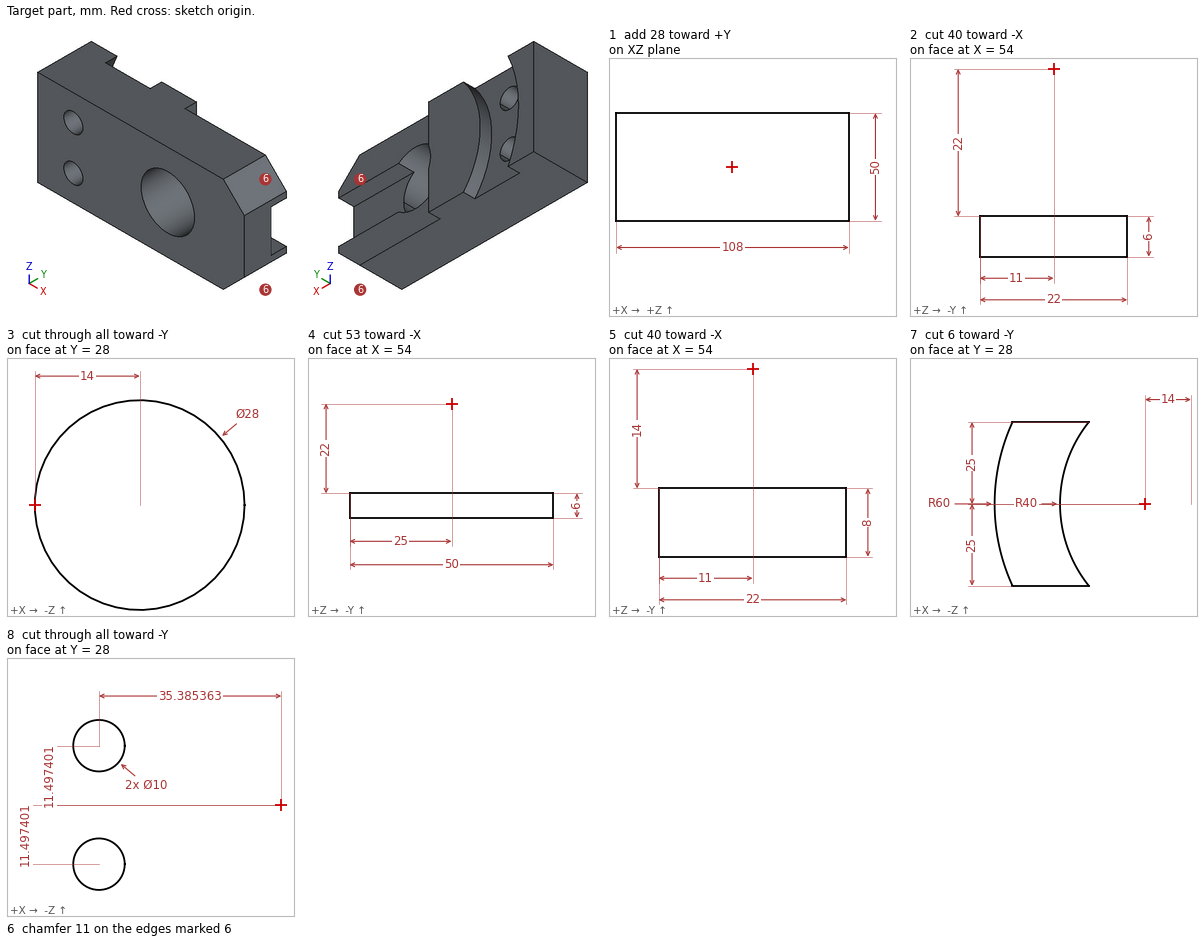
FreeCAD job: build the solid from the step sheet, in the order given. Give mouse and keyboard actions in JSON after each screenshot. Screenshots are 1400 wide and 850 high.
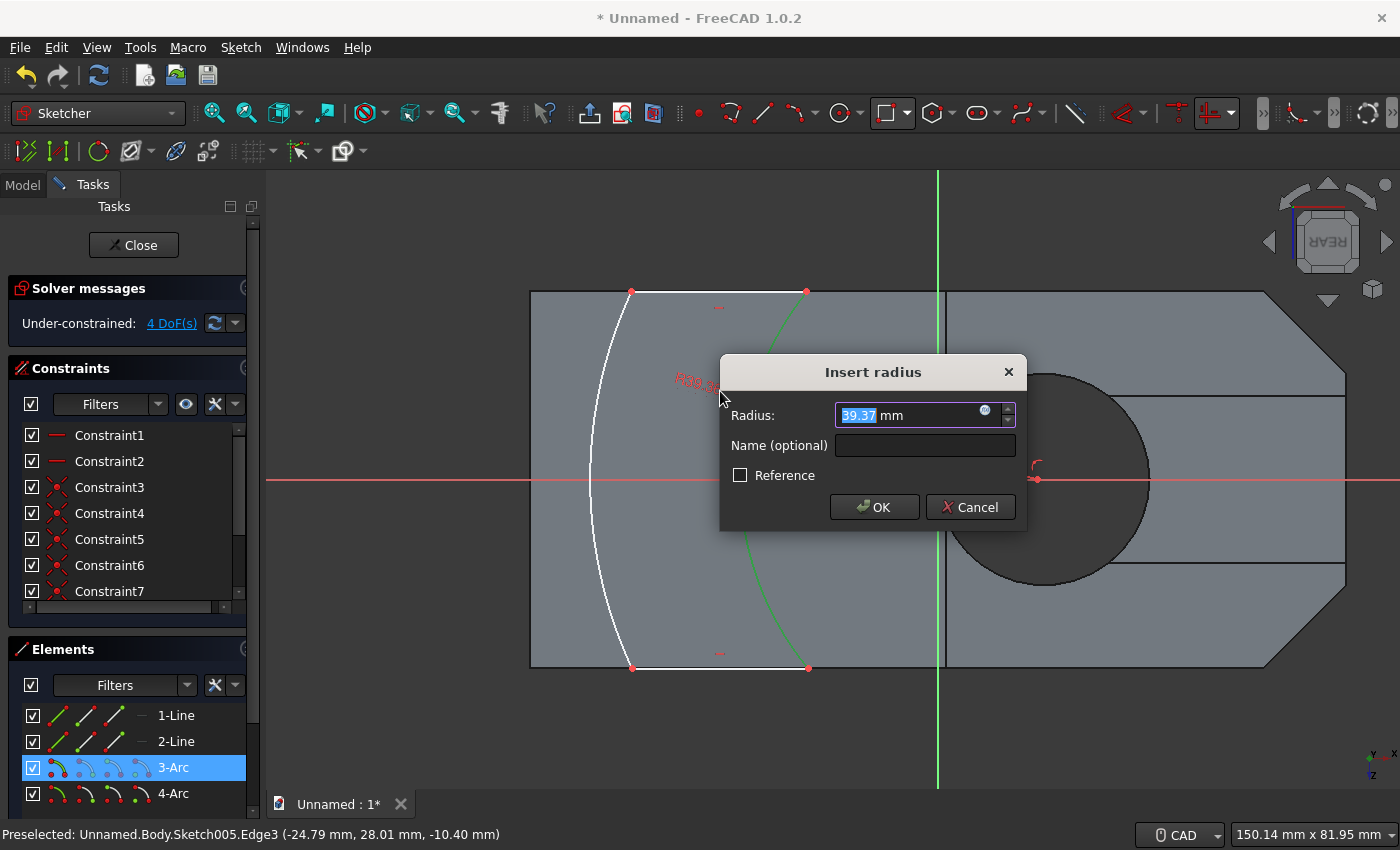
{"action": "type", "text": "40"}
{"action": "key", "text": "Return"}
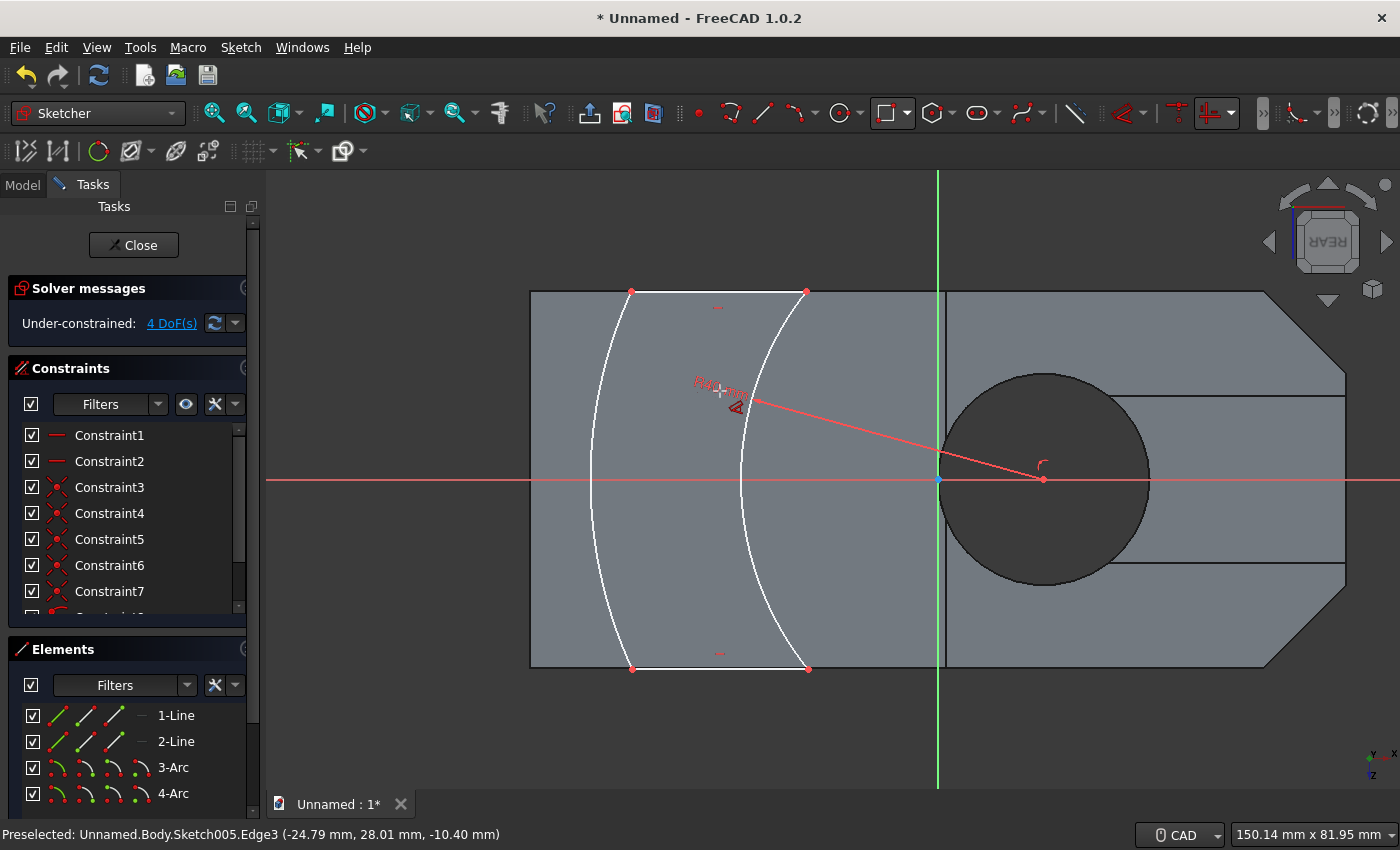
{"action": "left_click", "coordinate": [597, 403]}
{"action": "left_click", "coordinate": [565, 398]}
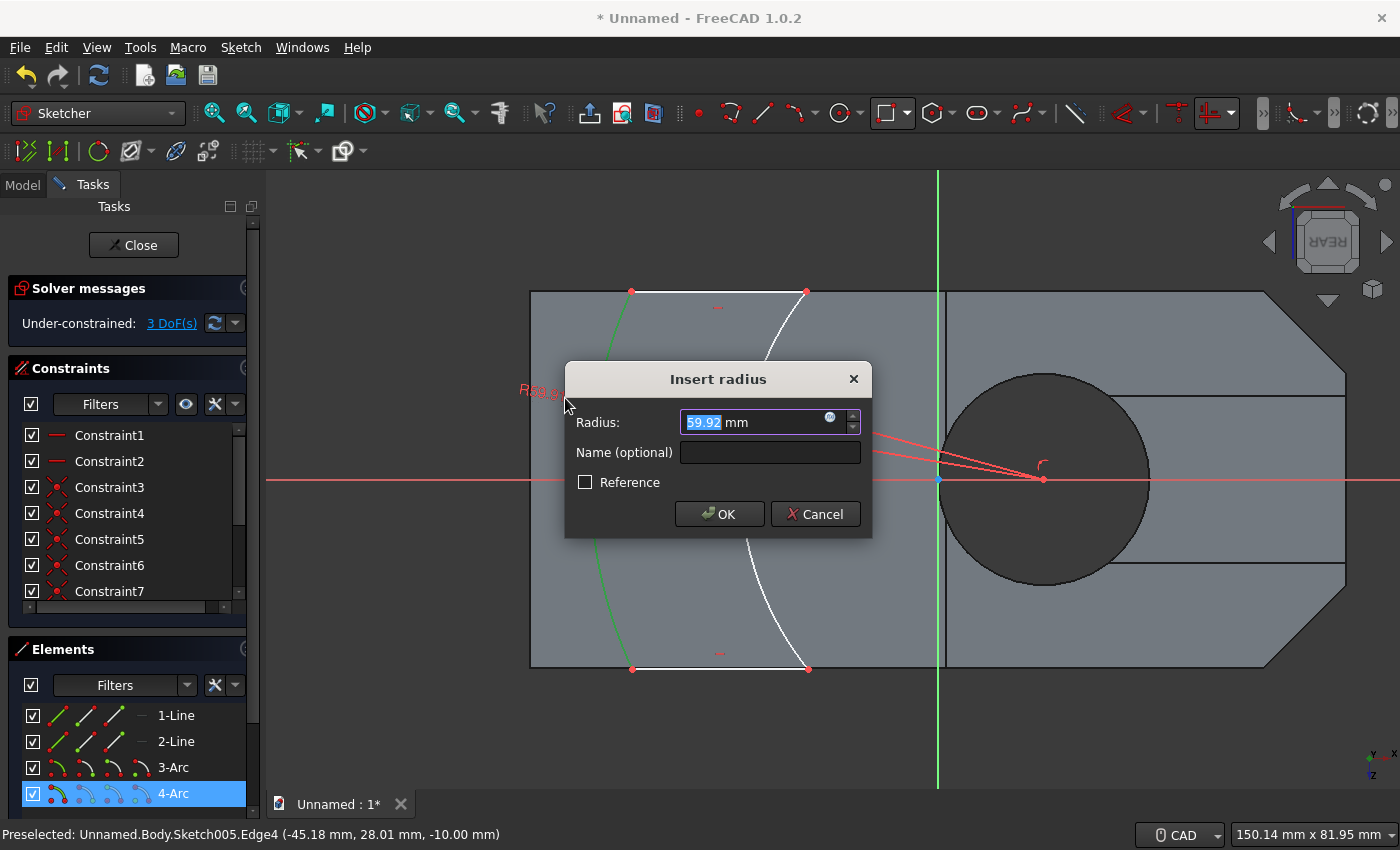
{"action": "type", "text": "60"}
{"action": "key", "text": "Return"}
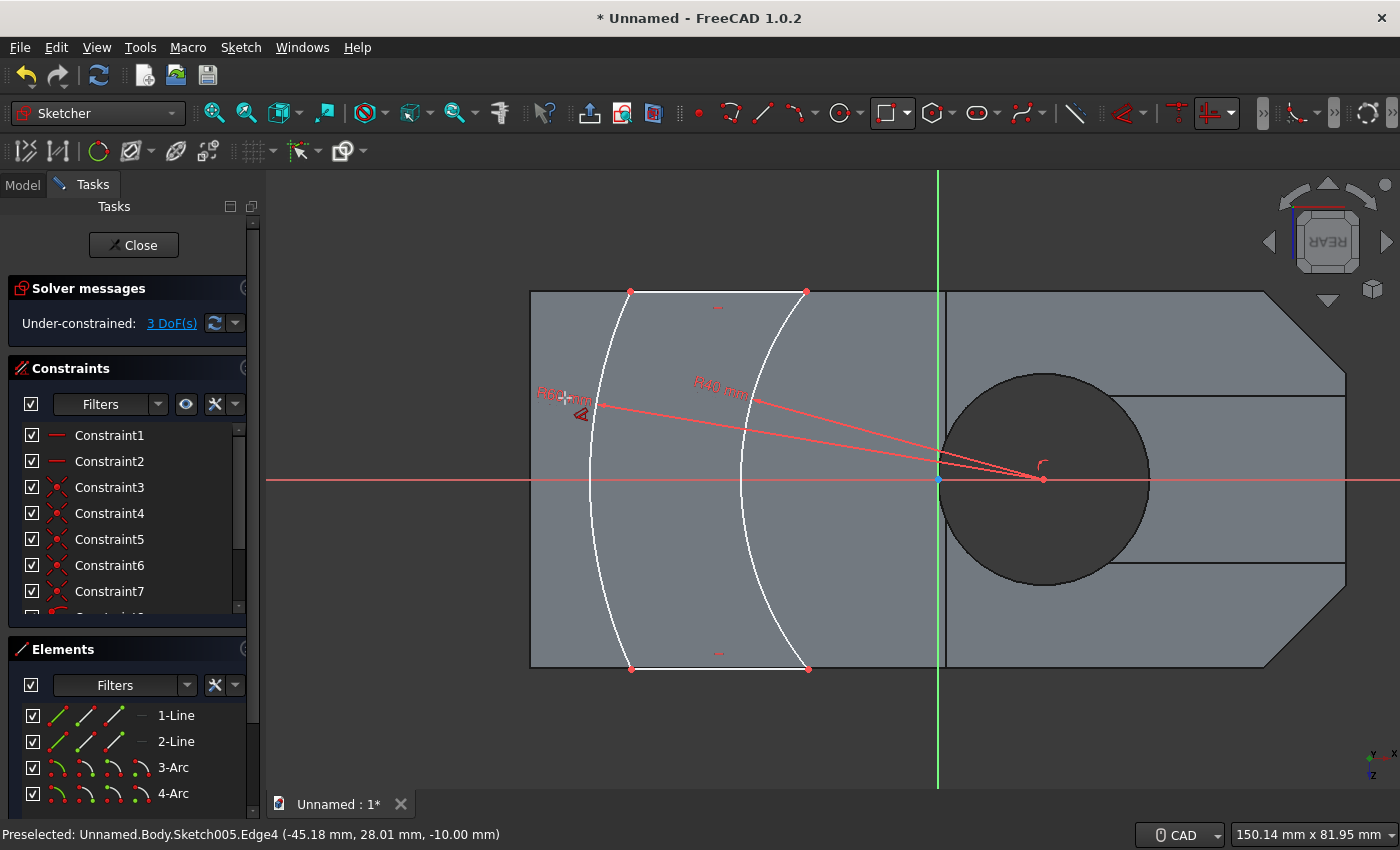
{"action": "left_click", "coordinate": [632, 669]}
{"action": "left_click", "coordinate": [972, 574]}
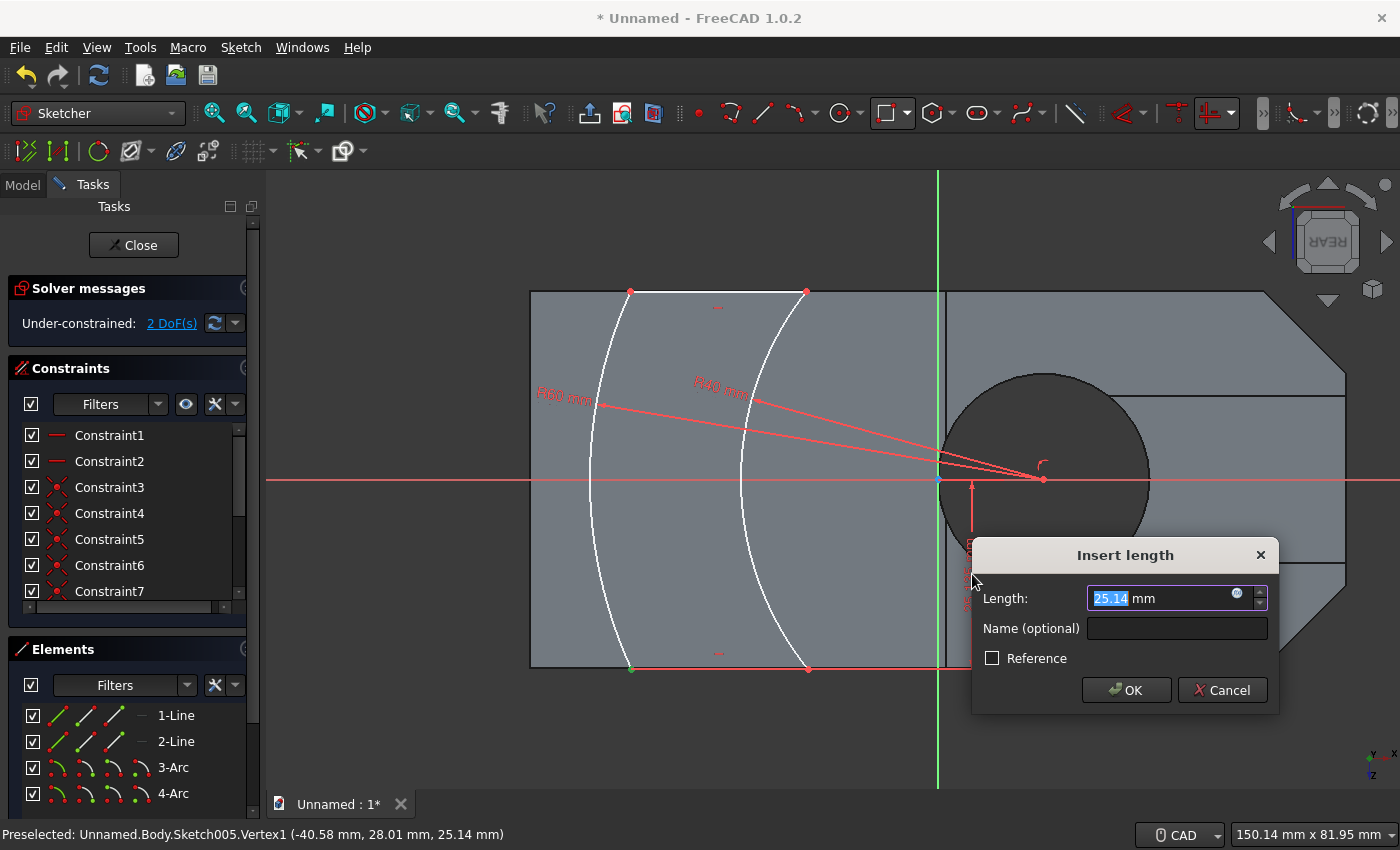
{"action": "type", "text": "25"}
{"action": "key", "text": "Return"}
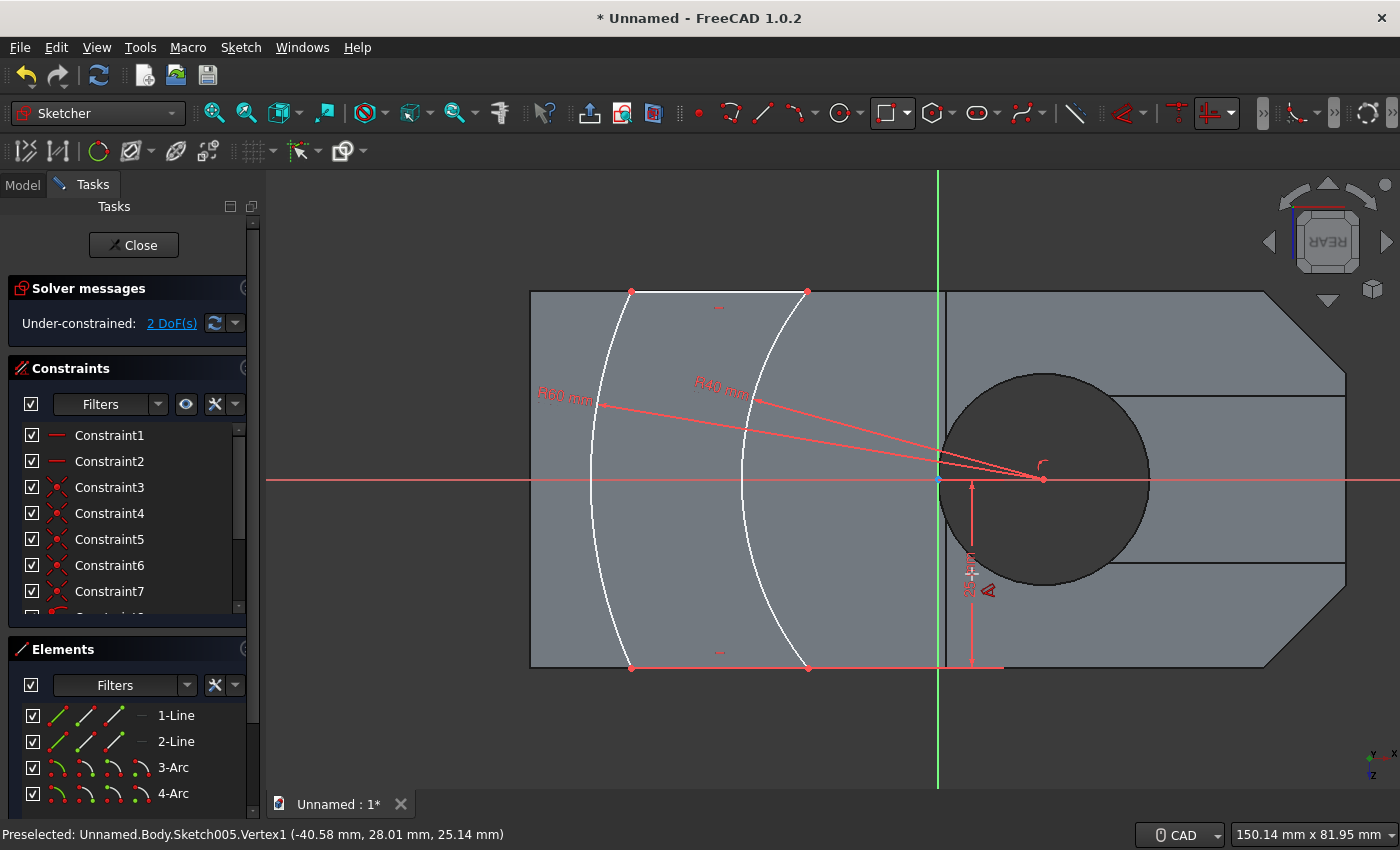
{"action": "left_click", "coordinate": [807, 292]}
{"action": "left_click", "coordinate": [972, 386]}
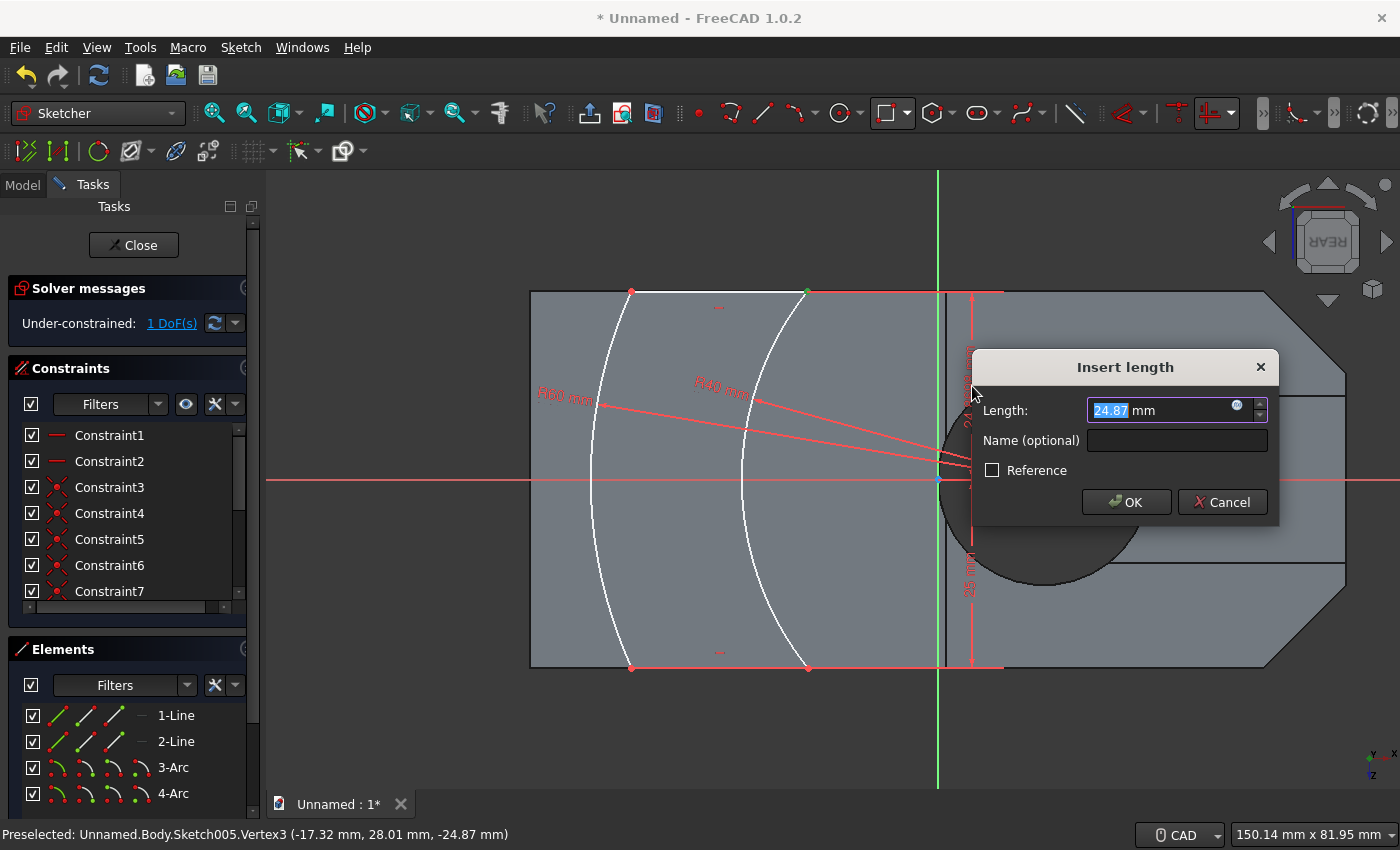
{"action": "type", "text": "25"}
{"action": "key", "text": "Return"}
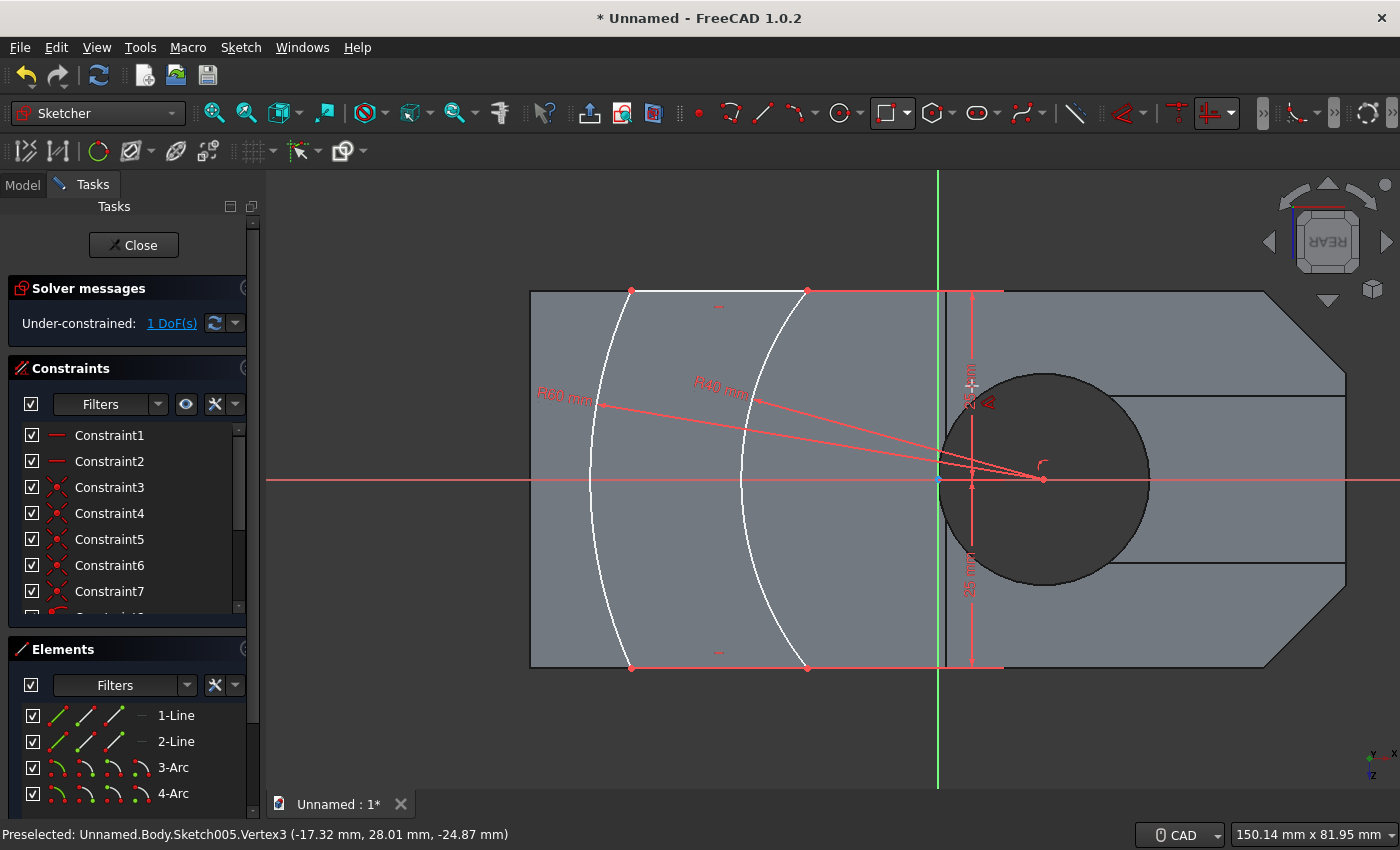
{"action": "left_click", "coordinate": [1043, 479]}
{"action": "left_click", "coordinate": [991, 513]}